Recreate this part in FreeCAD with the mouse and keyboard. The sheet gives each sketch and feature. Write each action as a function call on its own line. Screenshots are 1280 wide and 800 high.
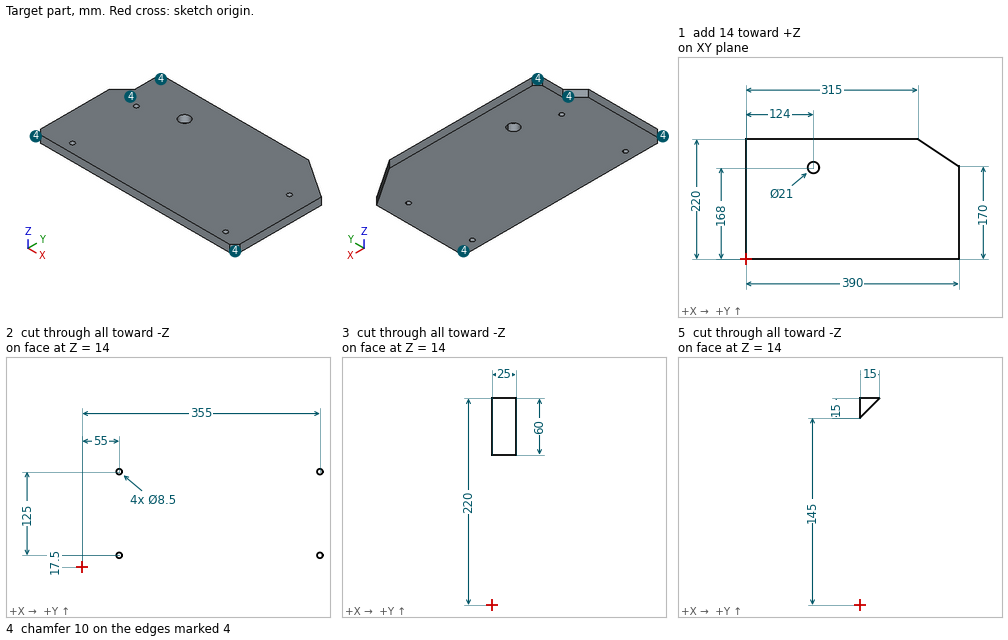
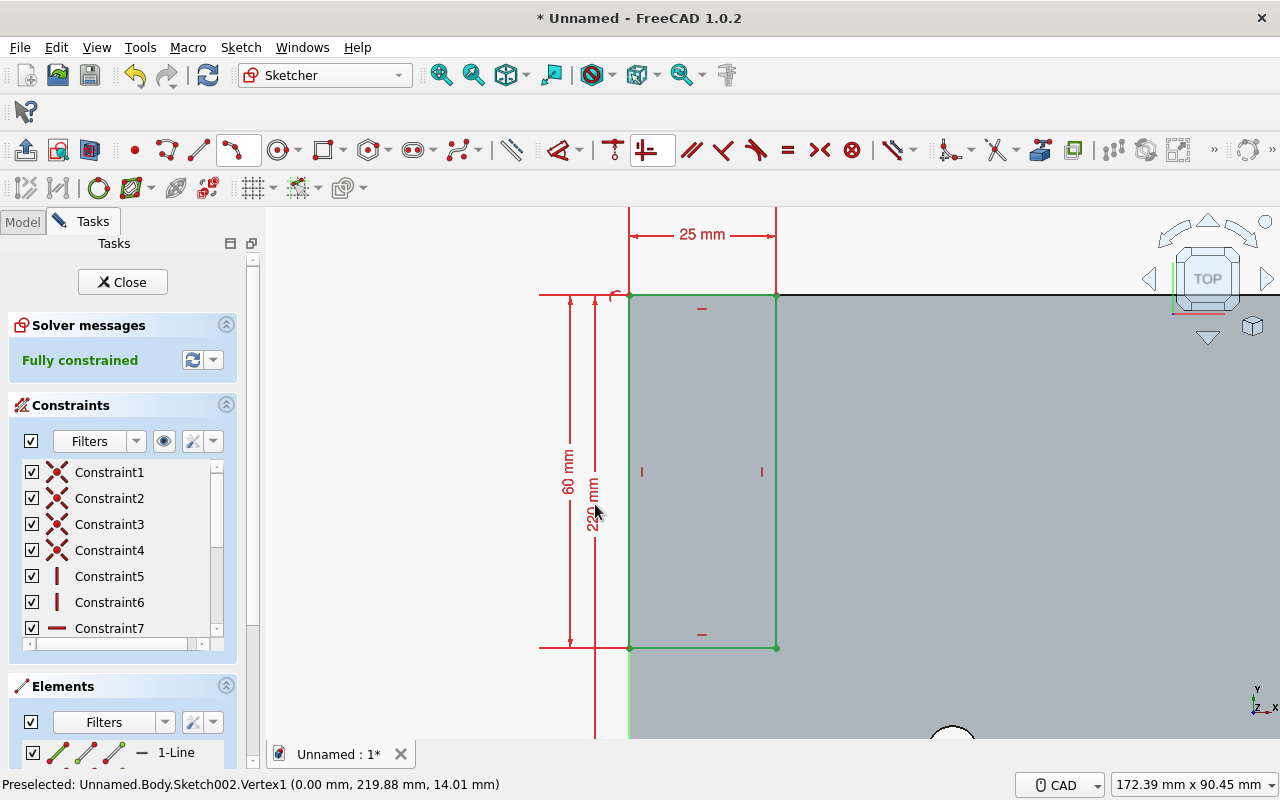
click(123, 282)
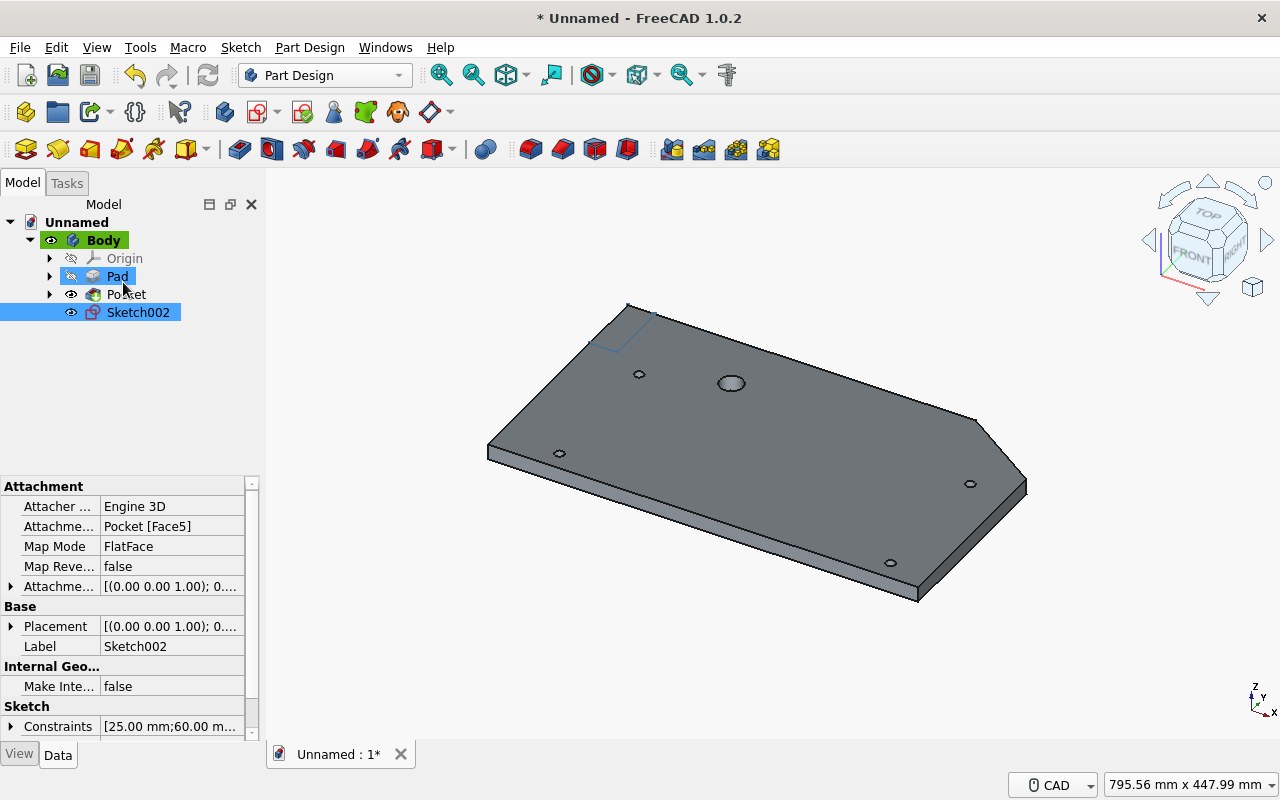
click(240, 150)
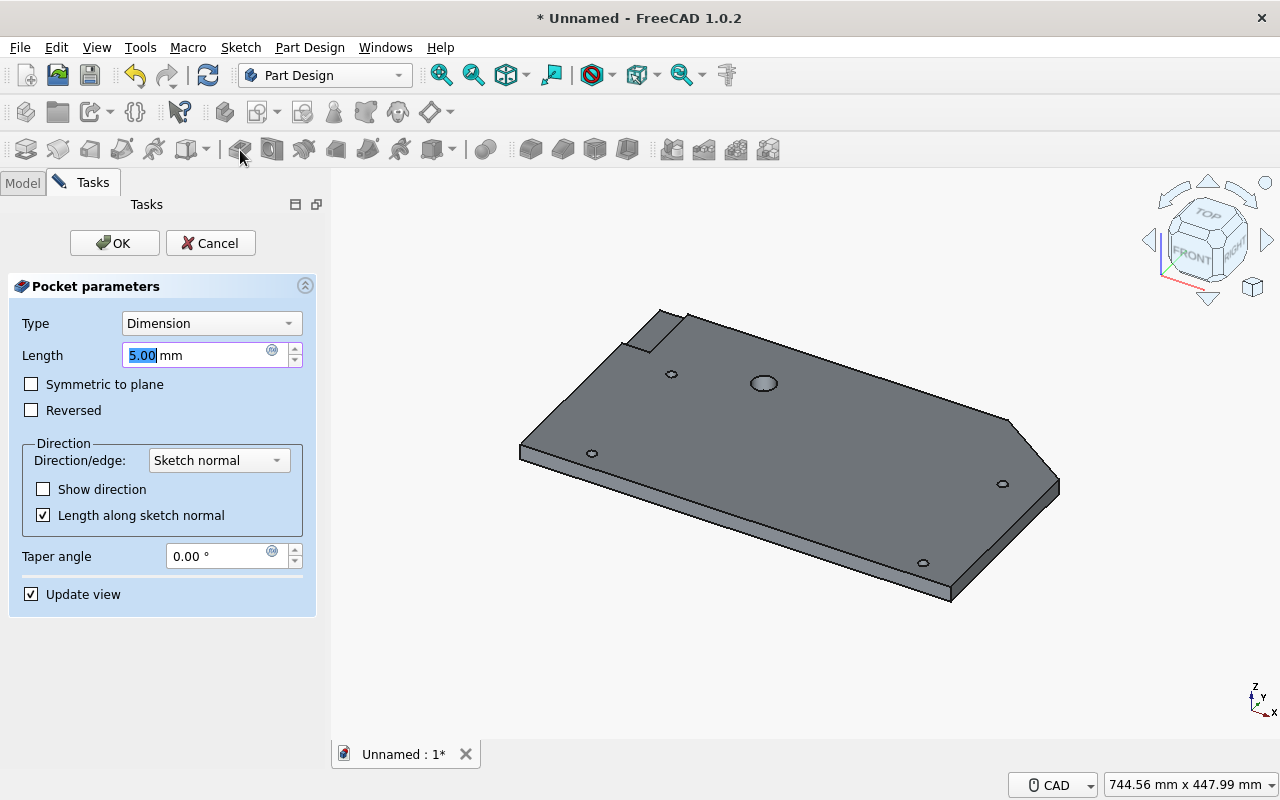
click(212, 324)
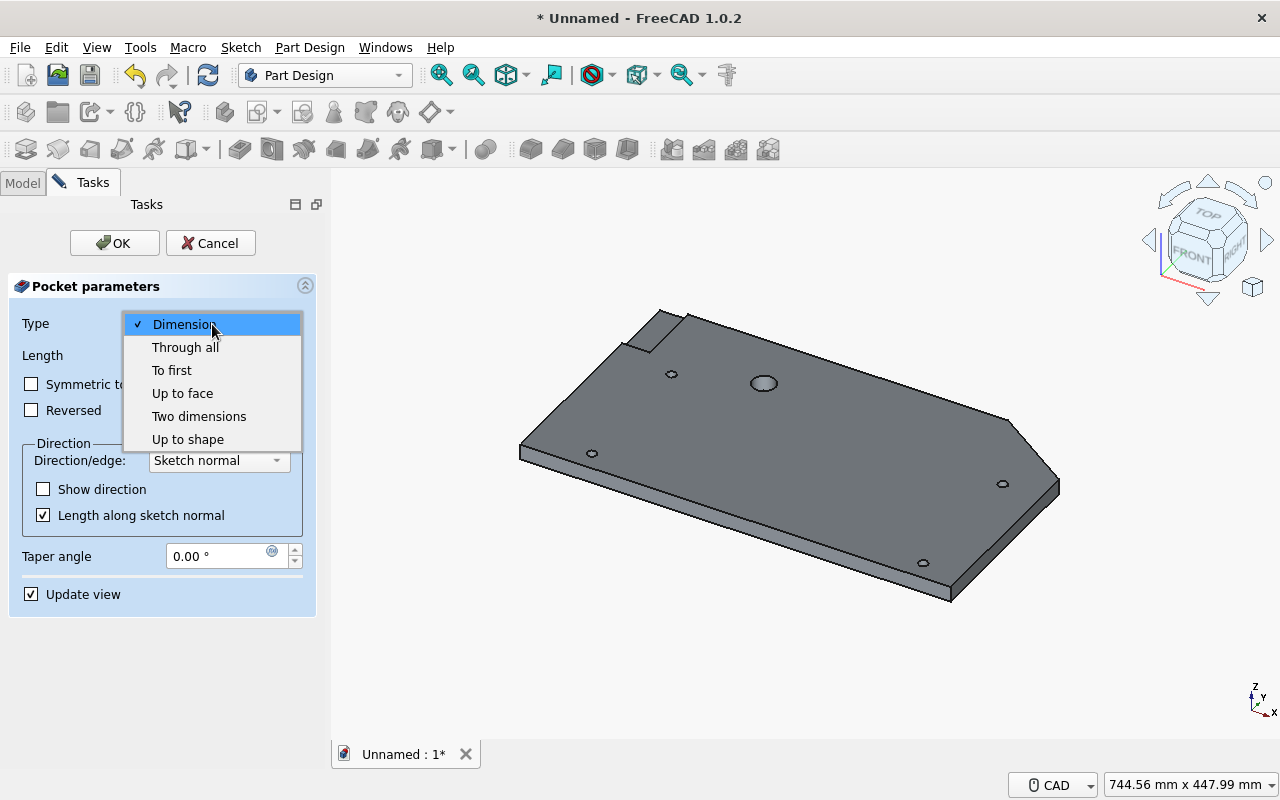
click(212, 348)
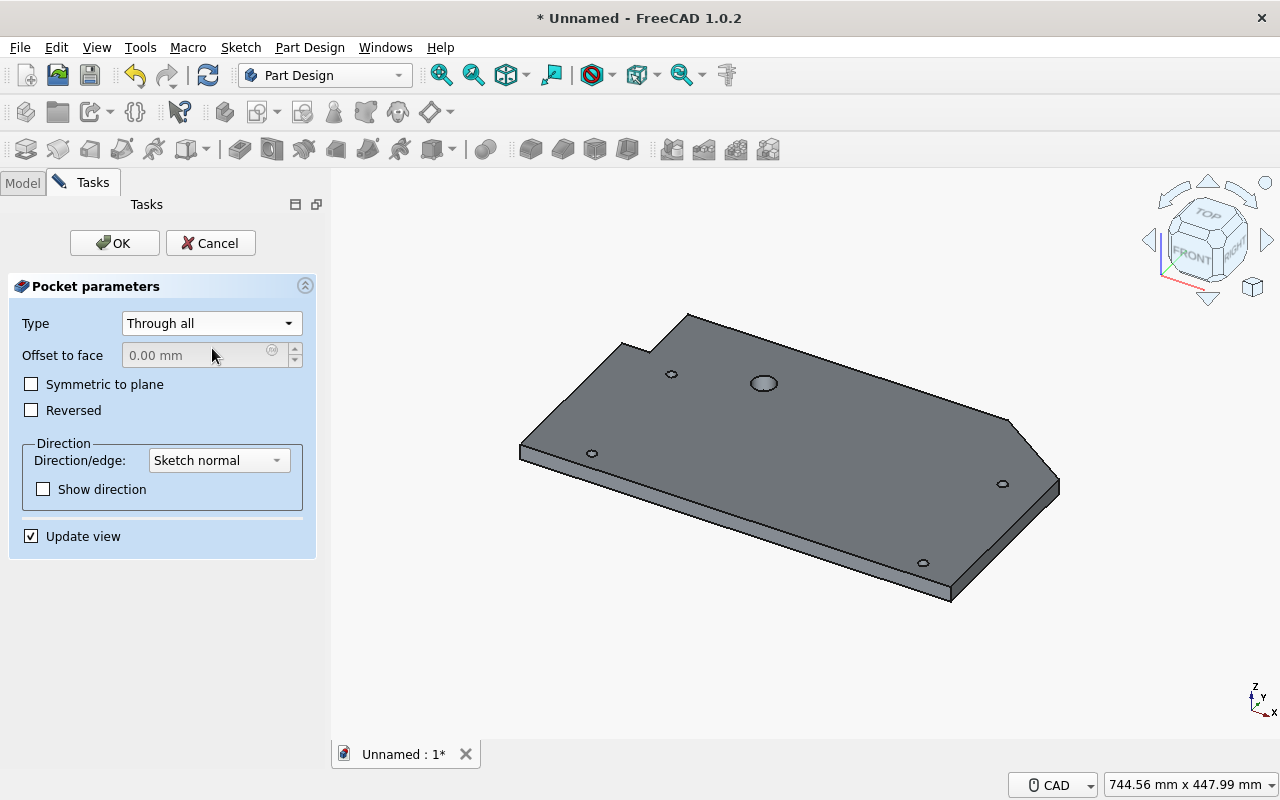
click(115, 243)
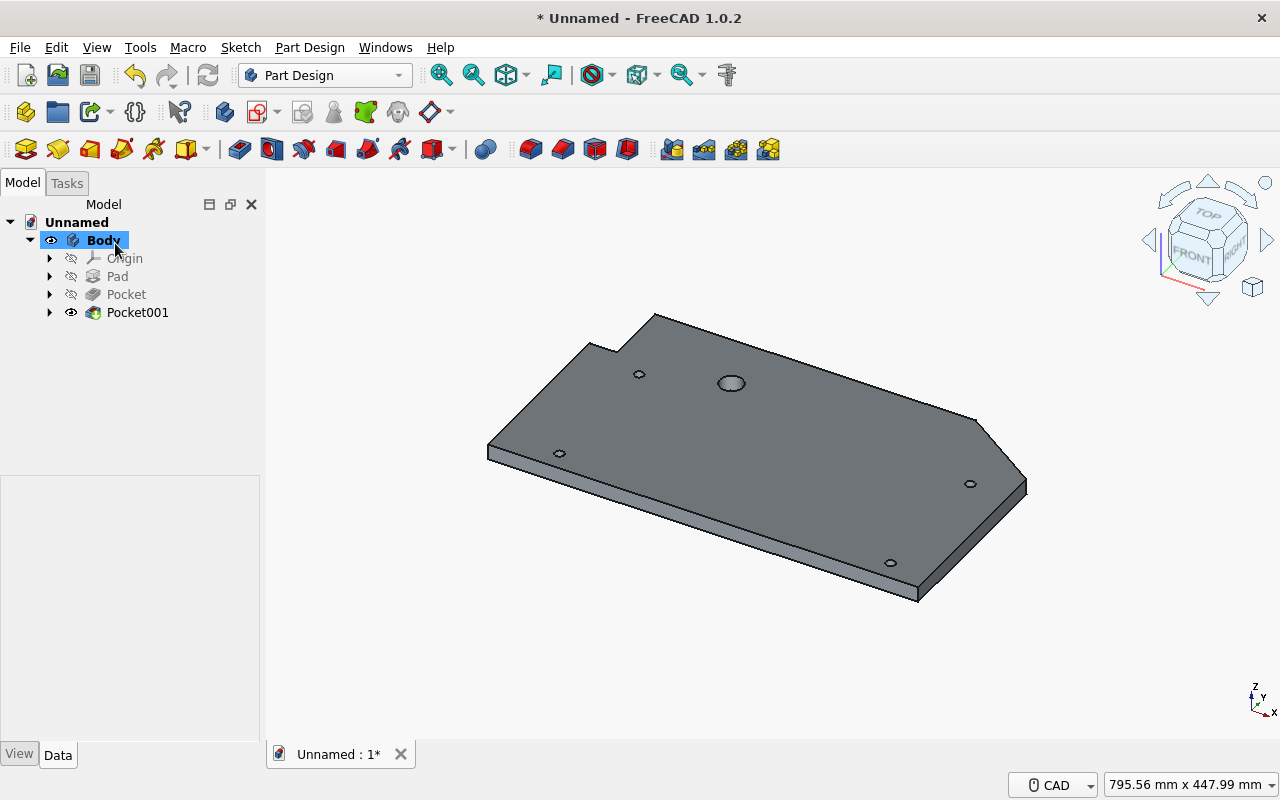
click(918, 593)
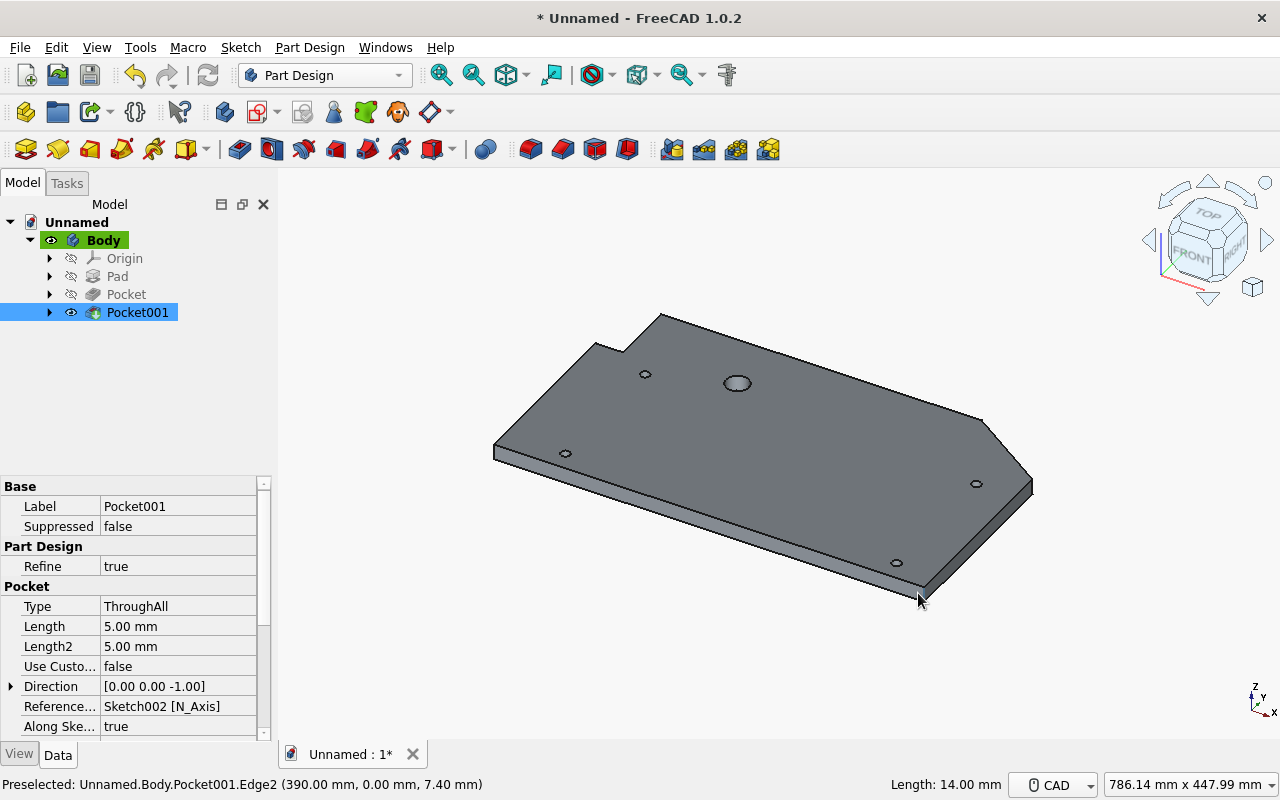
scroll(661, 321, up, 5)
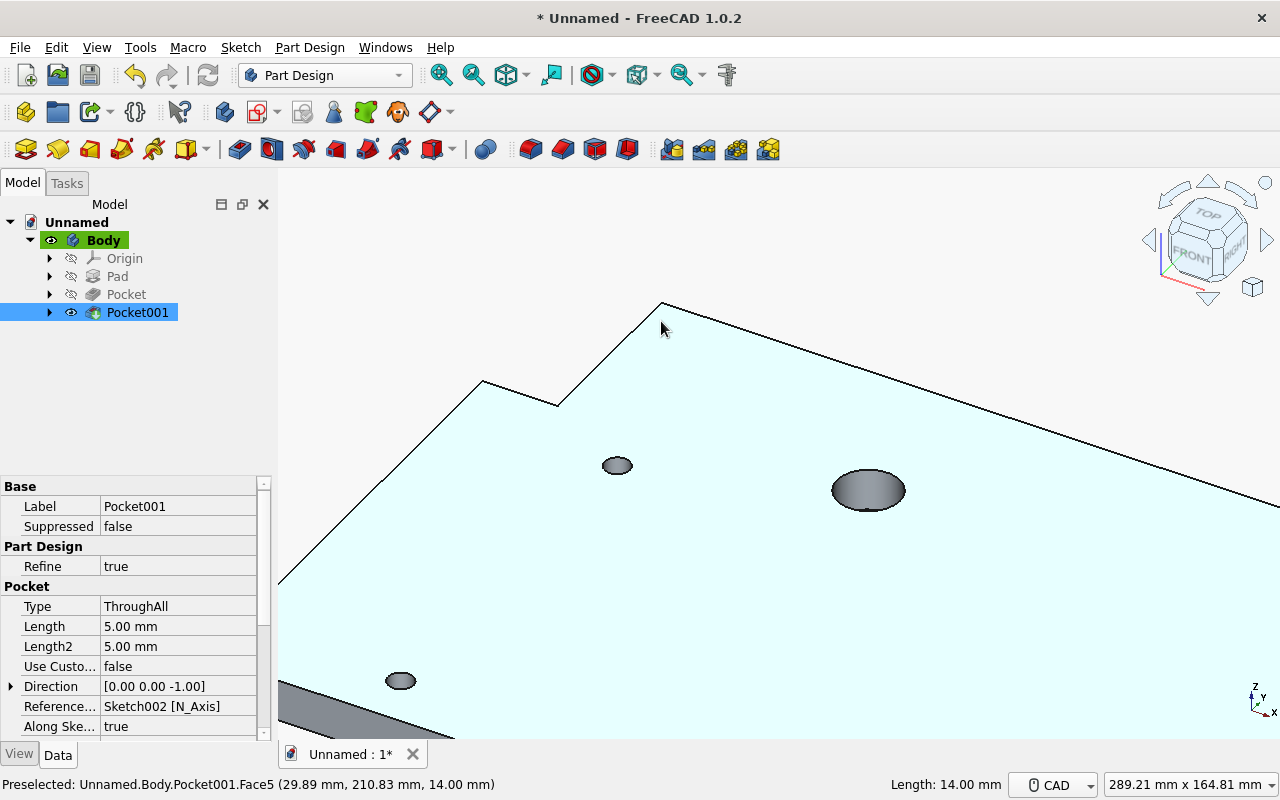
key(v)
key(f)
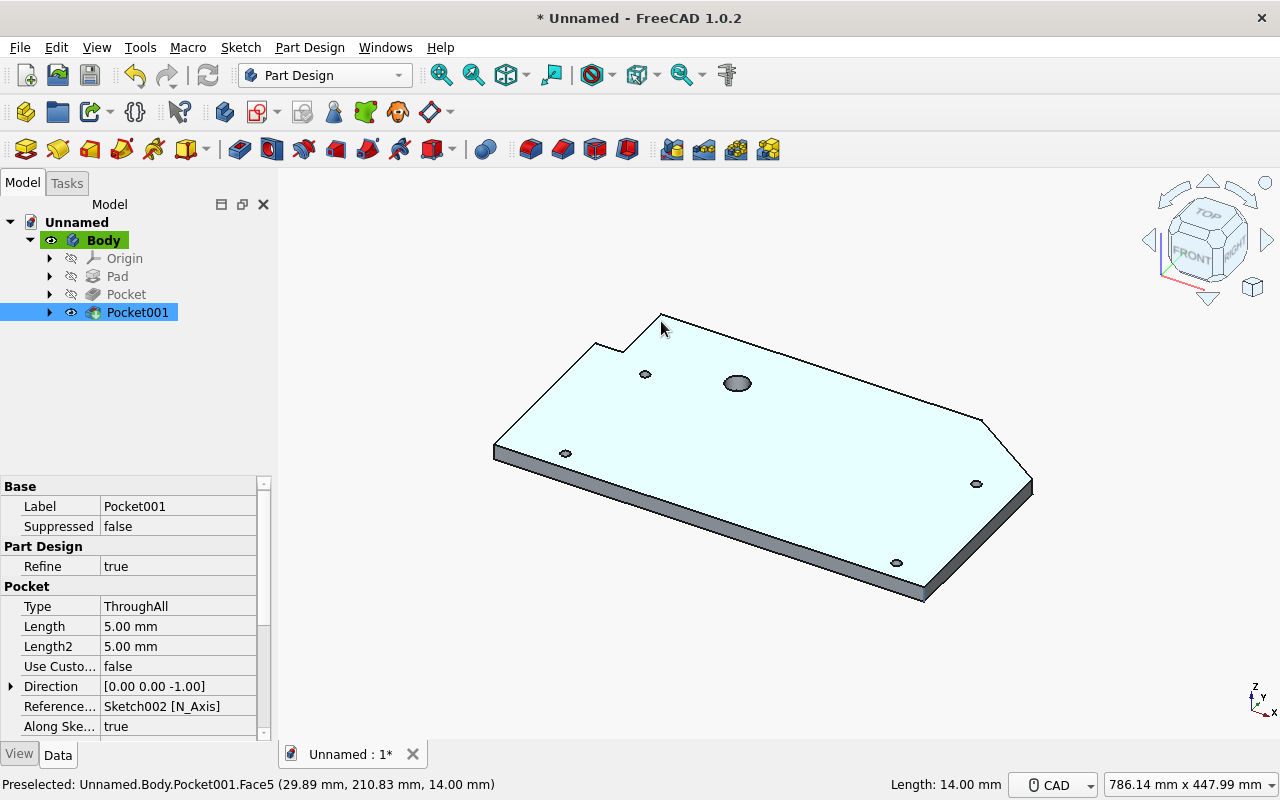
key(0)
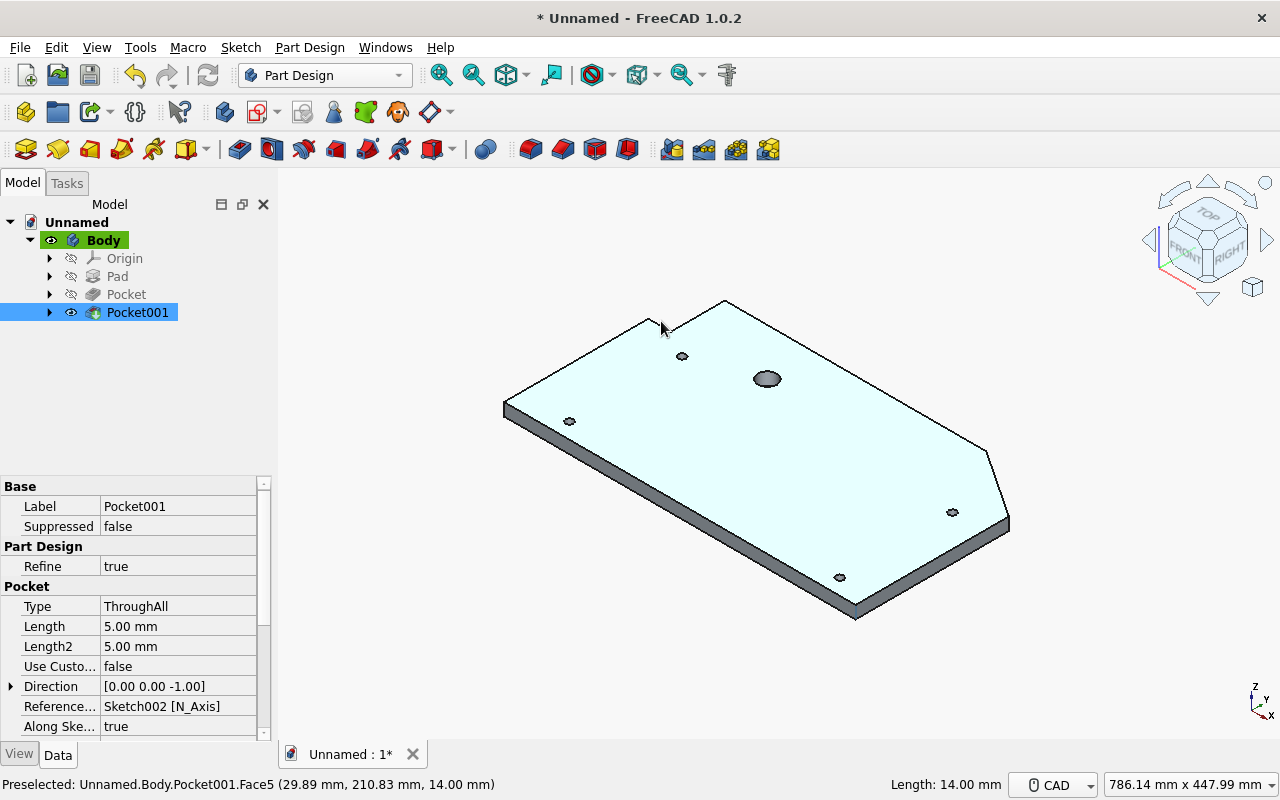
scroll(725, 307, up, 5)